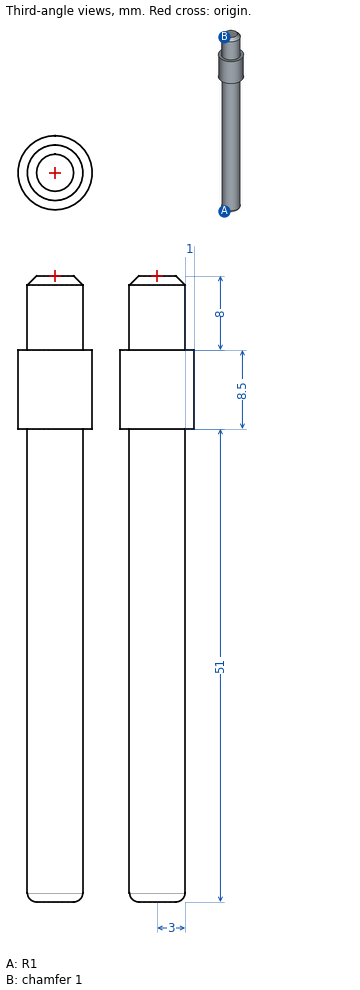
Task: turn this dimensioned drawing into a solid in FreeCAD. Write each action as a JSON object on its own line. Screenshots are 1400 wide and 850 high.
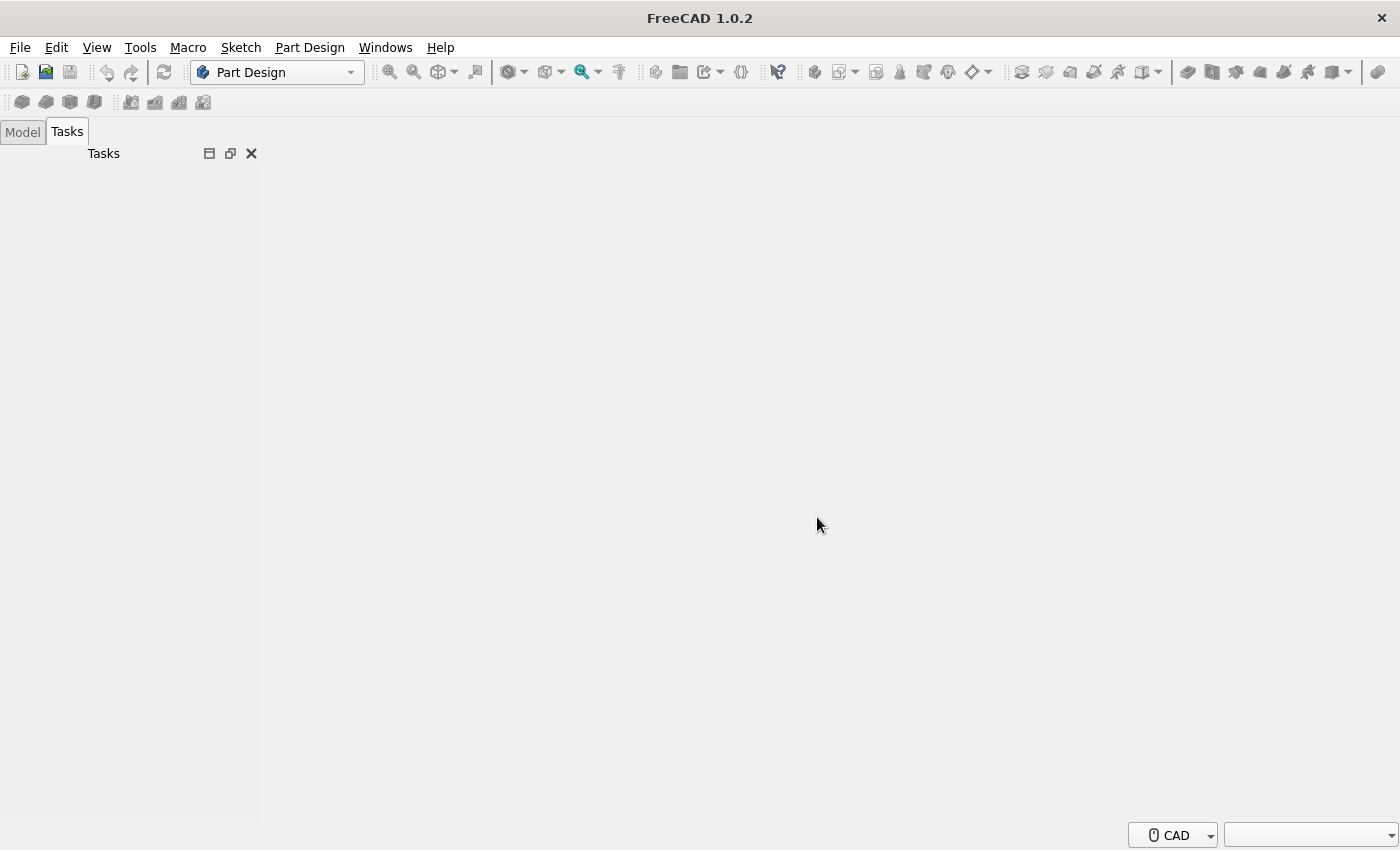
{"action": "left_click", "coordinate": [22, 72]}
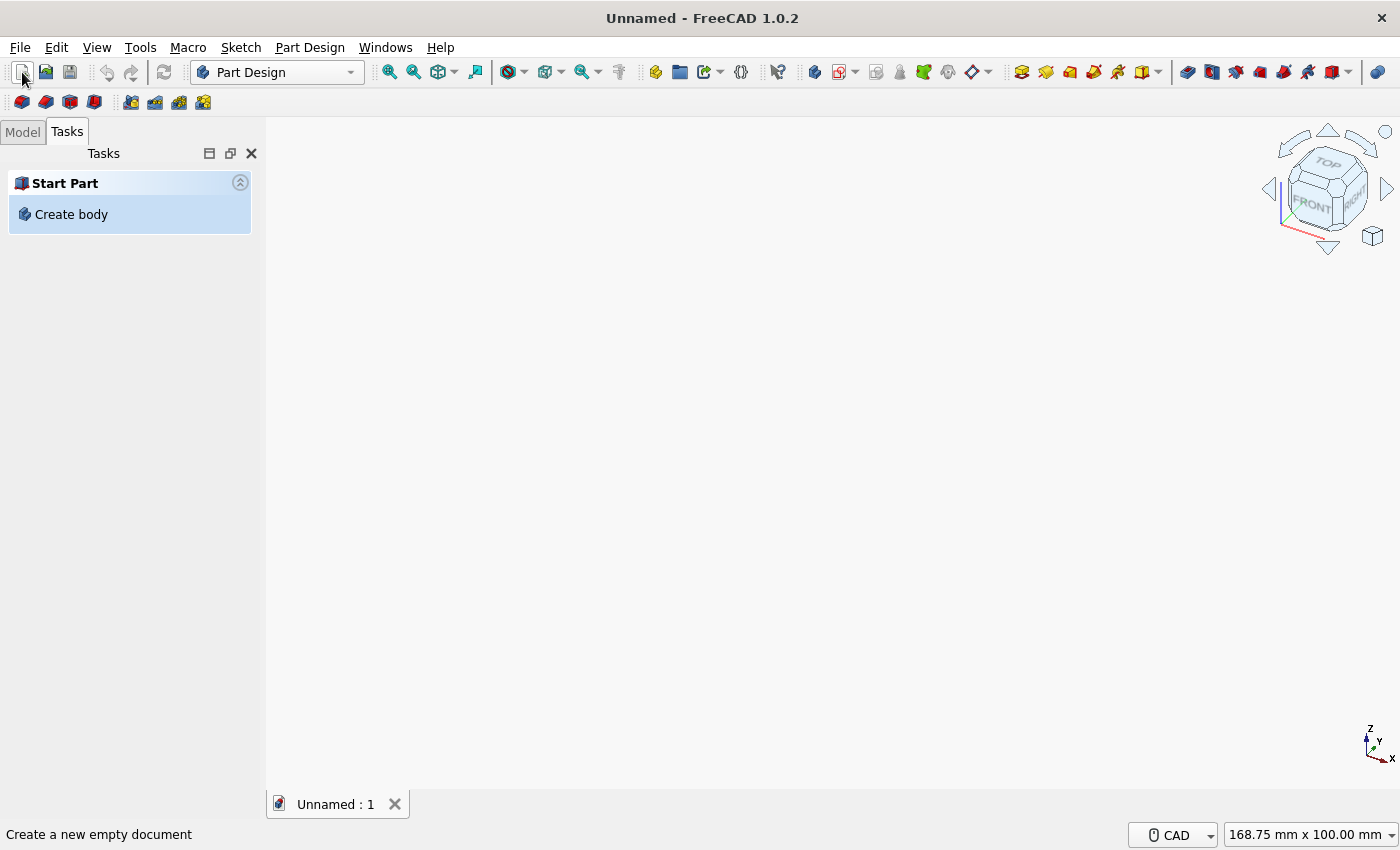
{"action": "left_click", "coordinate": [840, 72]}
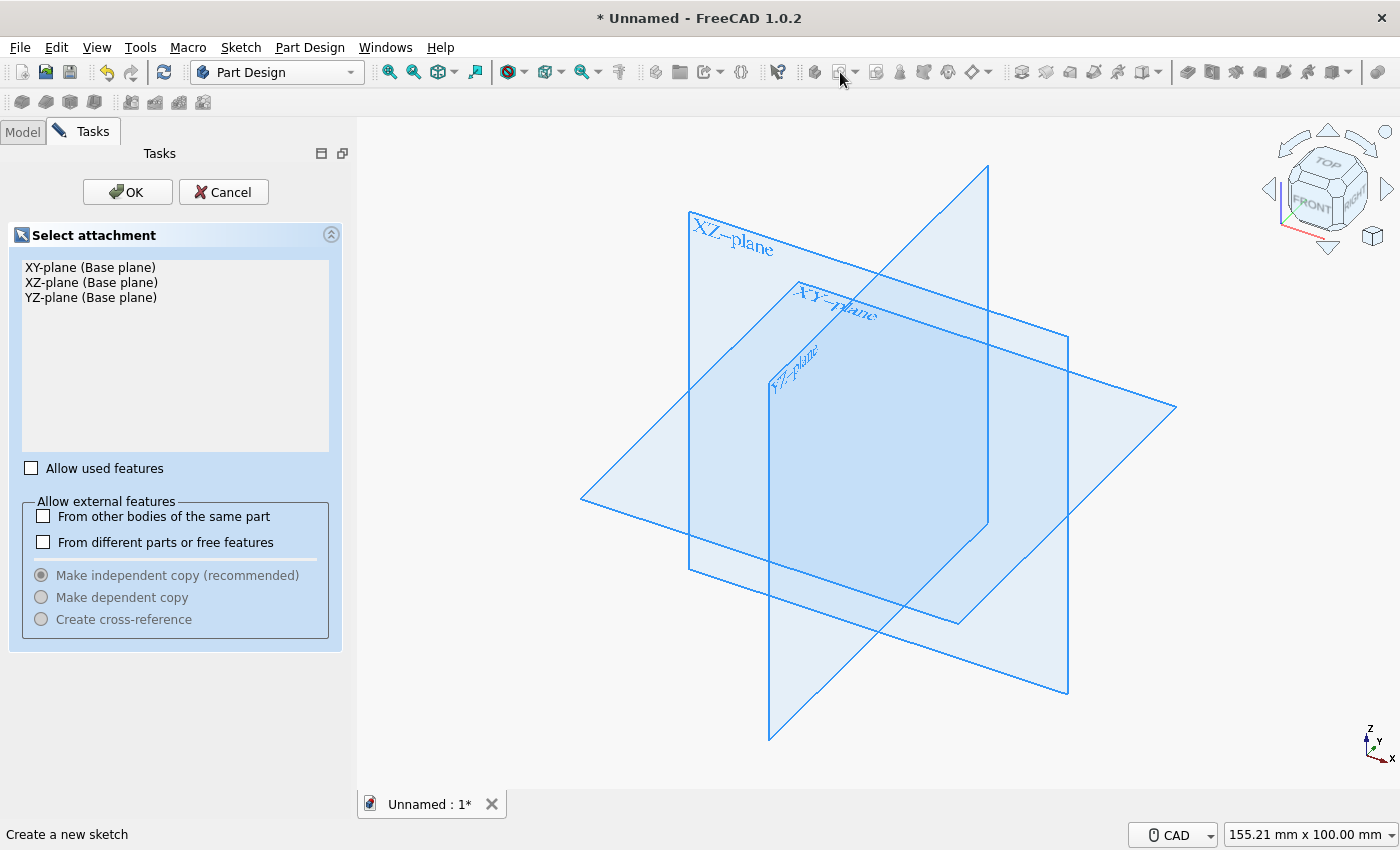
{"action": "left_click", "coordinate": [82, 298]}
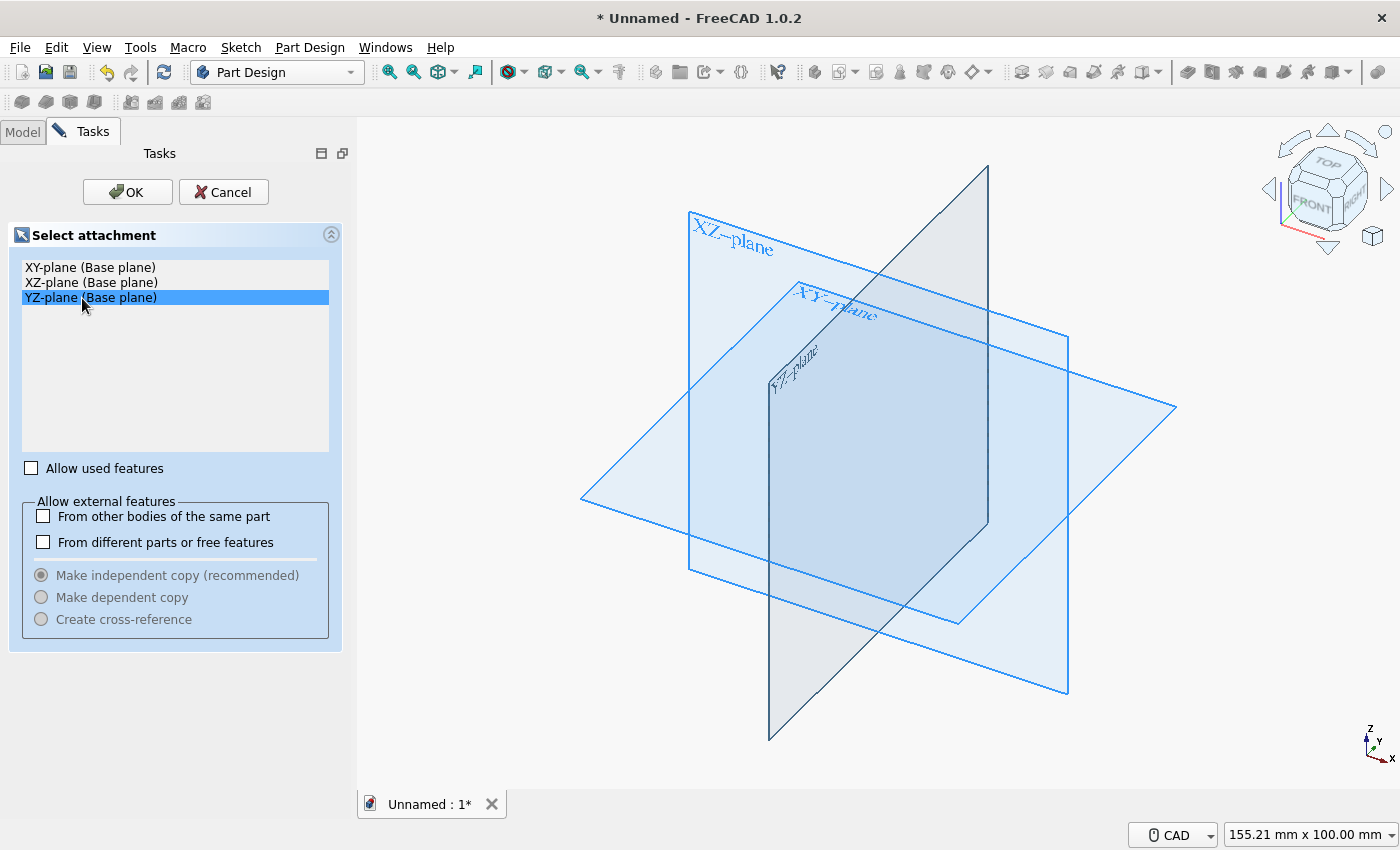
{"action": "left_click", "coordinate": [128, 192]}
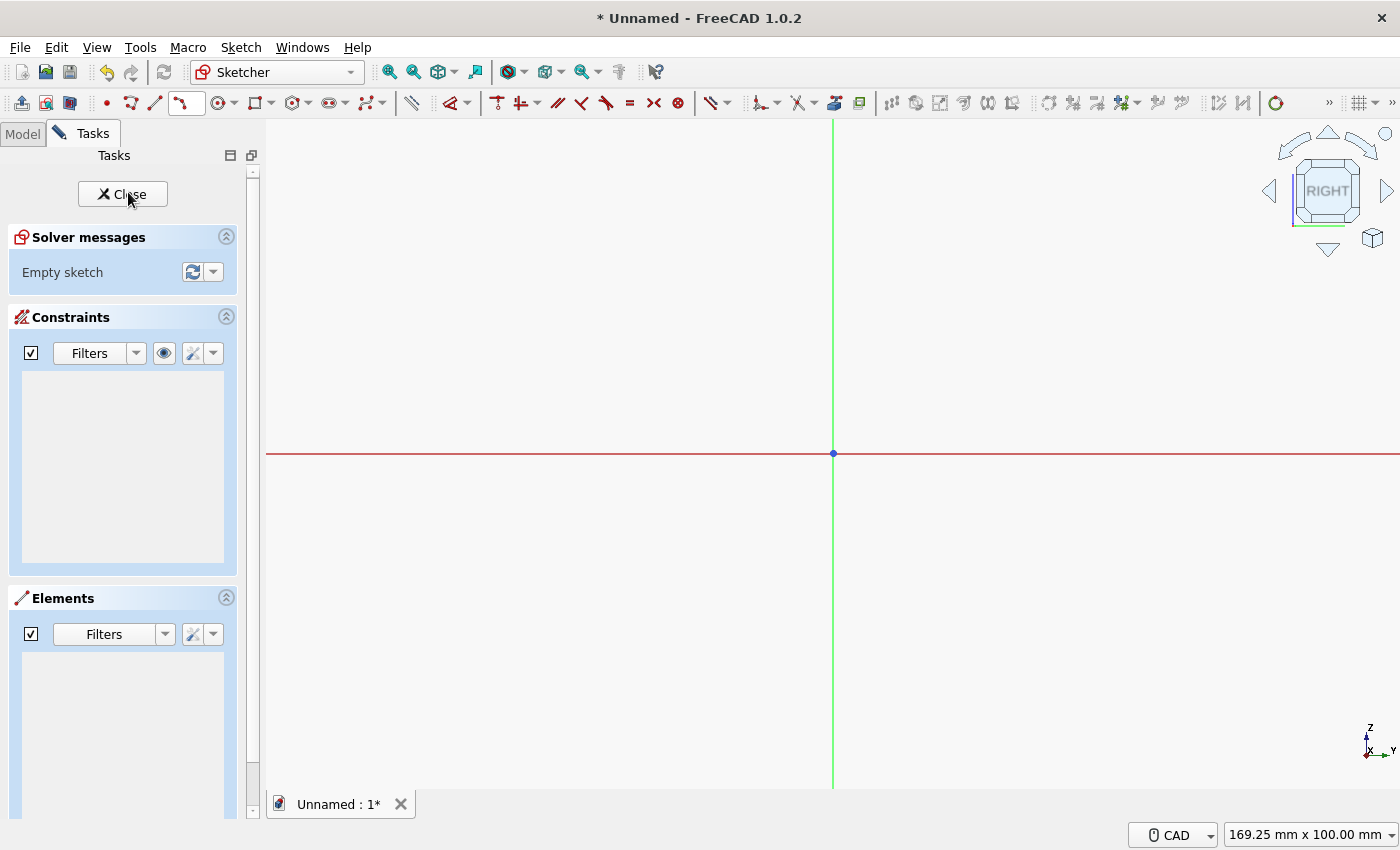
{"action": "scroll", "coordinate": [598, 147], "scroll_direction": "down", "scroll_amount": 2}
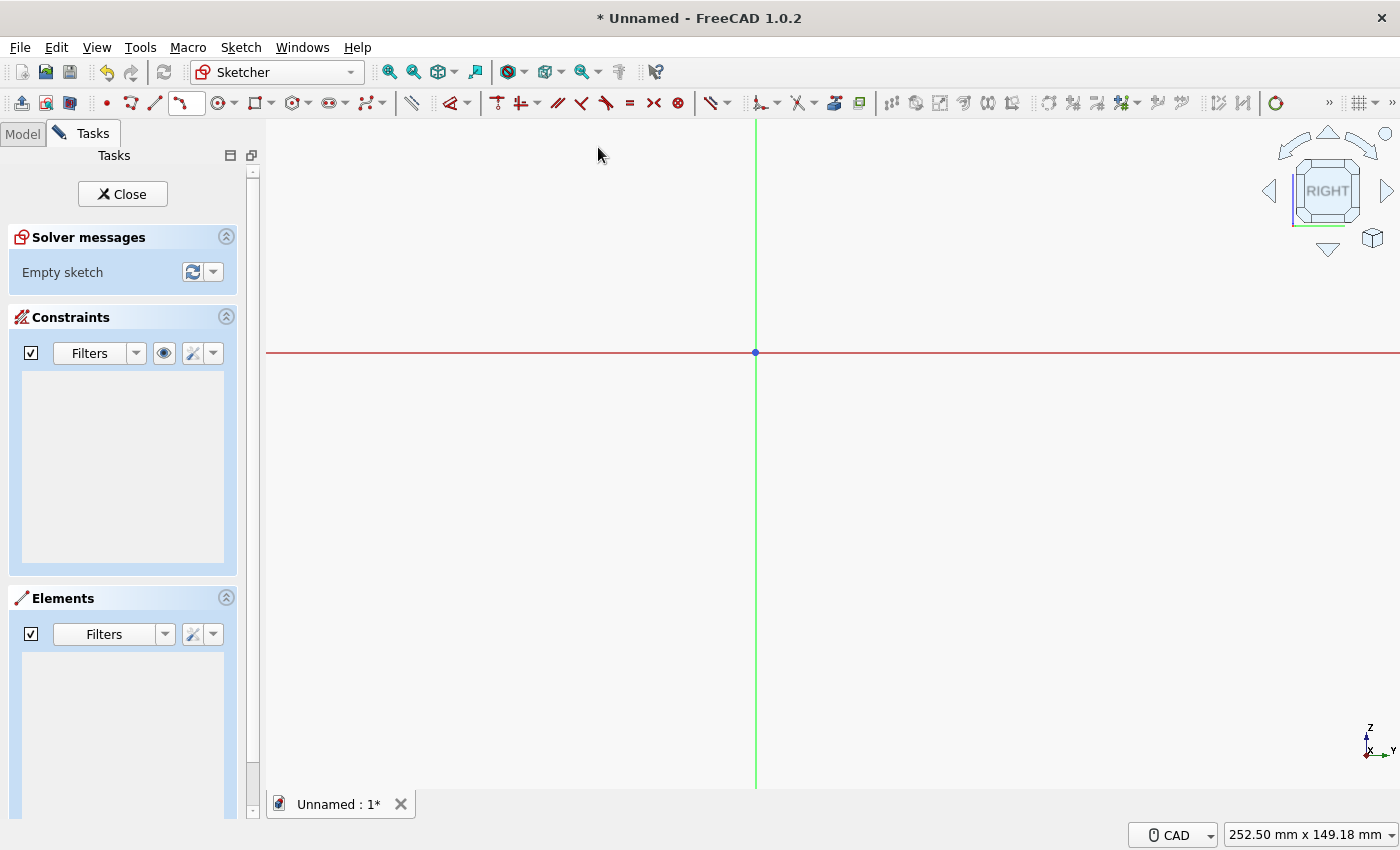
{"action": "scroll", "coordinate": [765, 607], "scroll_direction": "up", "scroll_amount": 2}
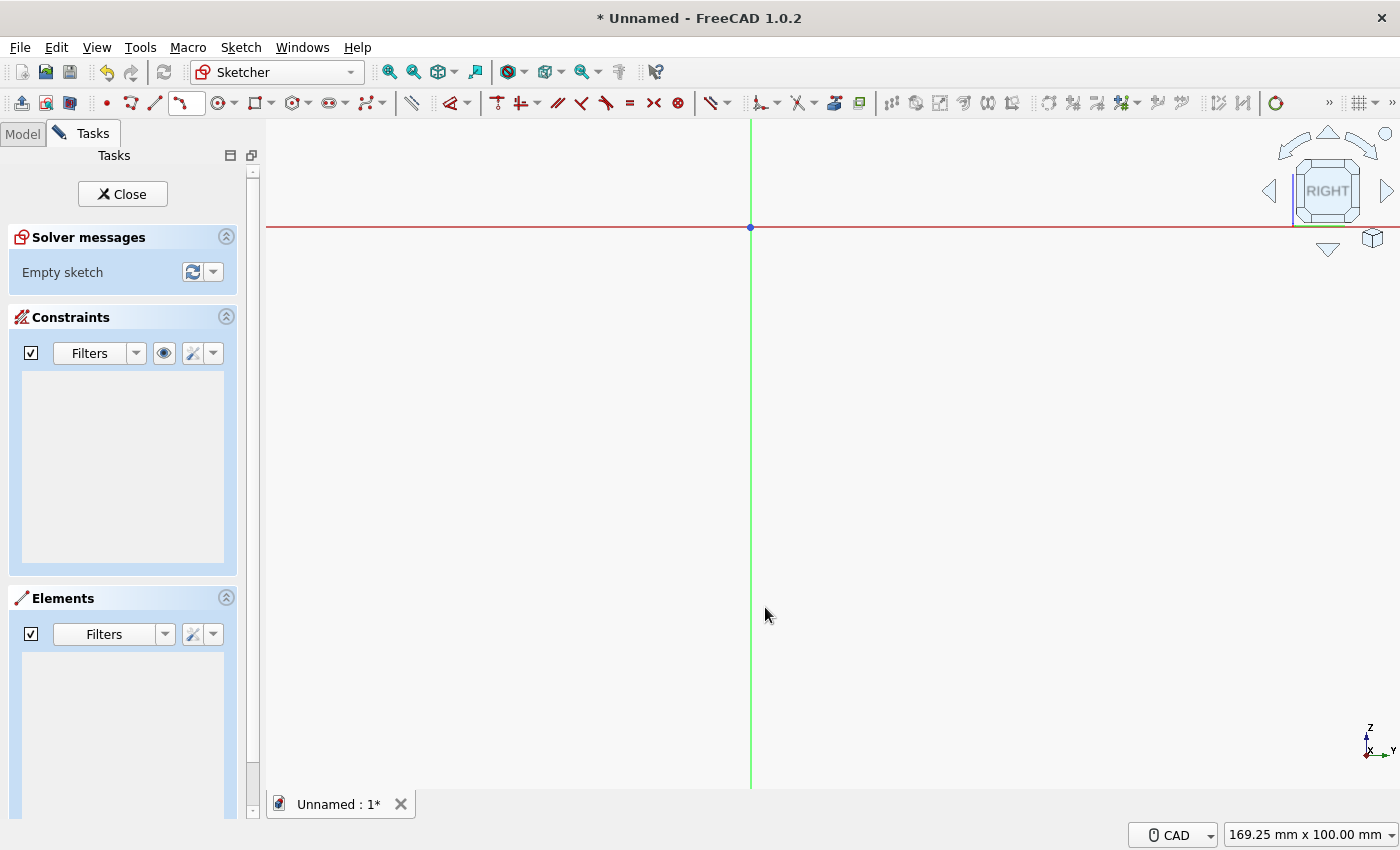
{"action": "left_click", "coordinate": [132, 104]}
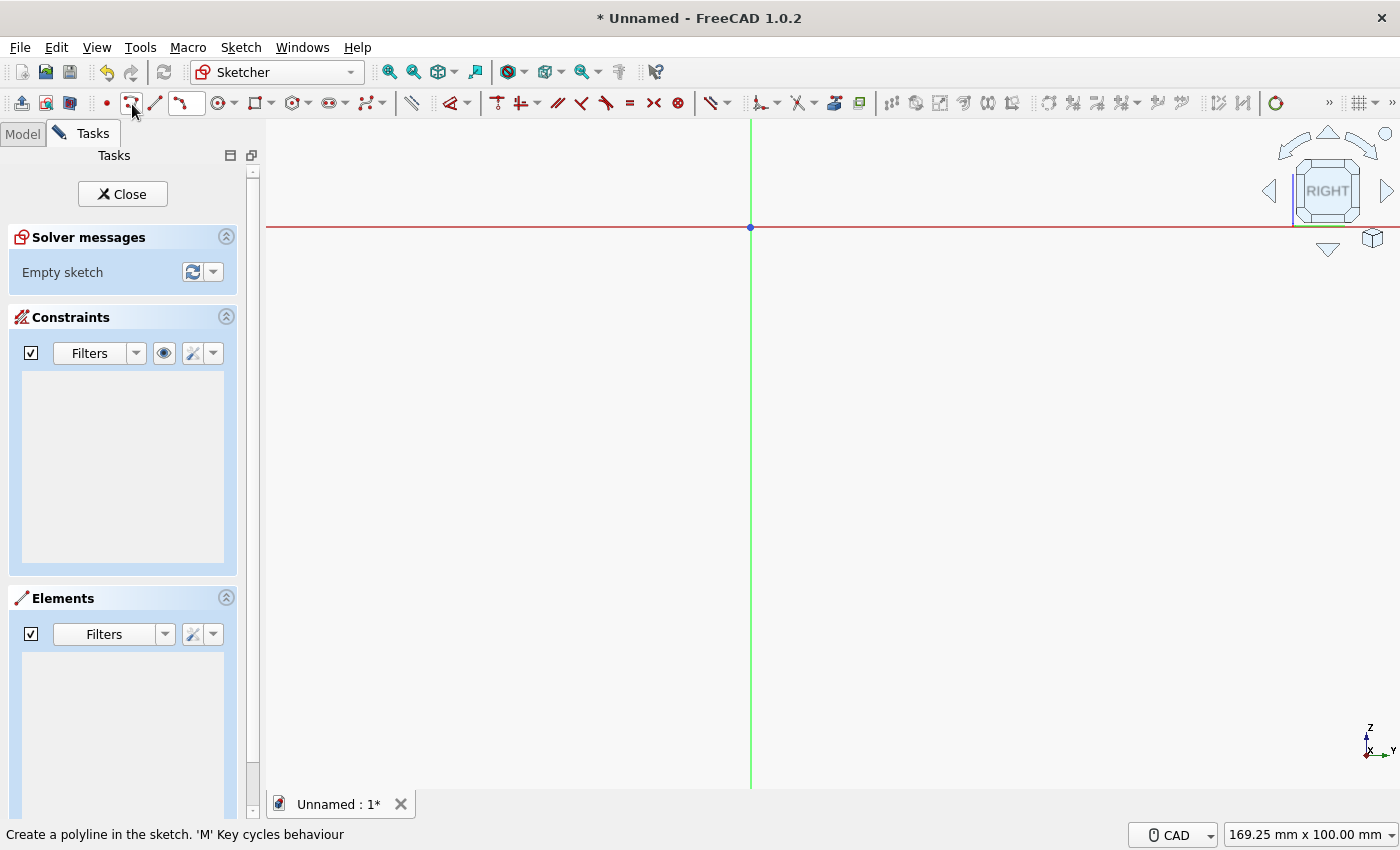
{"action": "left_click", "coordinate": [751, 227]}
{"action": "left_click", "coordinate": [760, 680]}
{"action": "left_click", "coordinate": [771, 680]}
{"action": "left_click", "coordinate": [771, 338]}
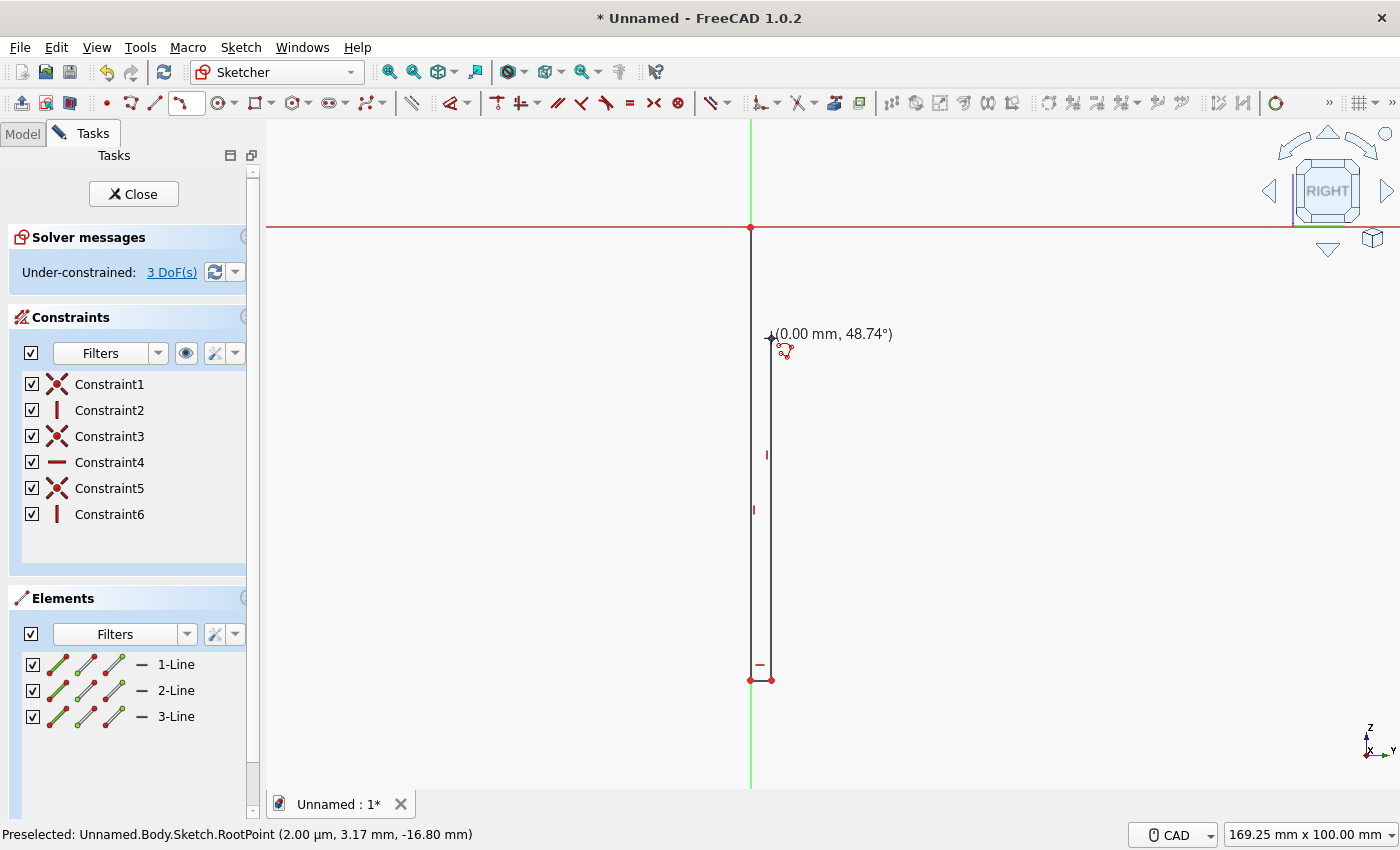
{"action": "scroll", "coordinate": [778, 338], "scroll_direction": "up", "scroll_amount": 5}